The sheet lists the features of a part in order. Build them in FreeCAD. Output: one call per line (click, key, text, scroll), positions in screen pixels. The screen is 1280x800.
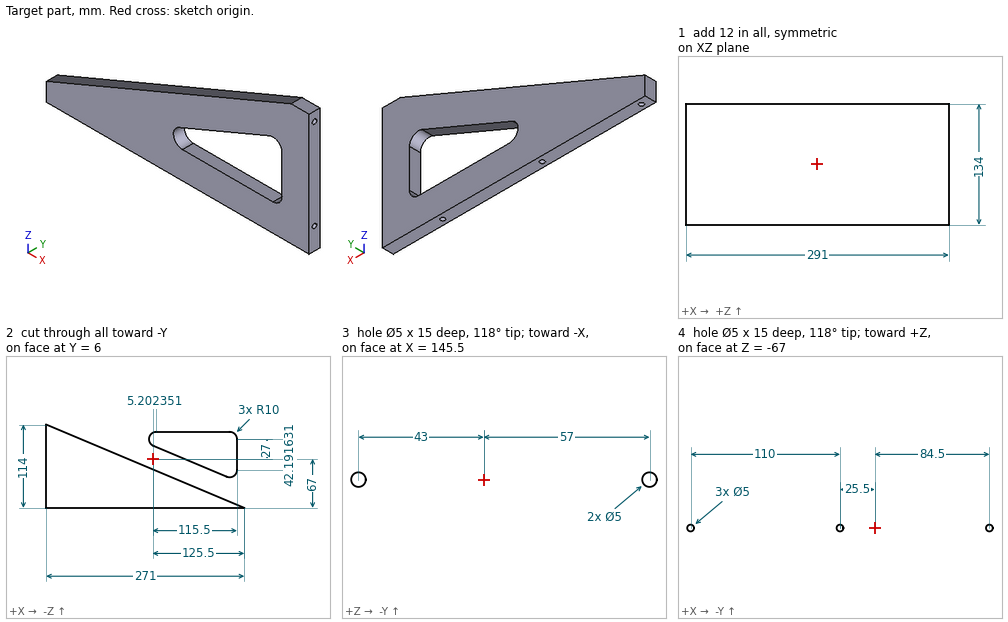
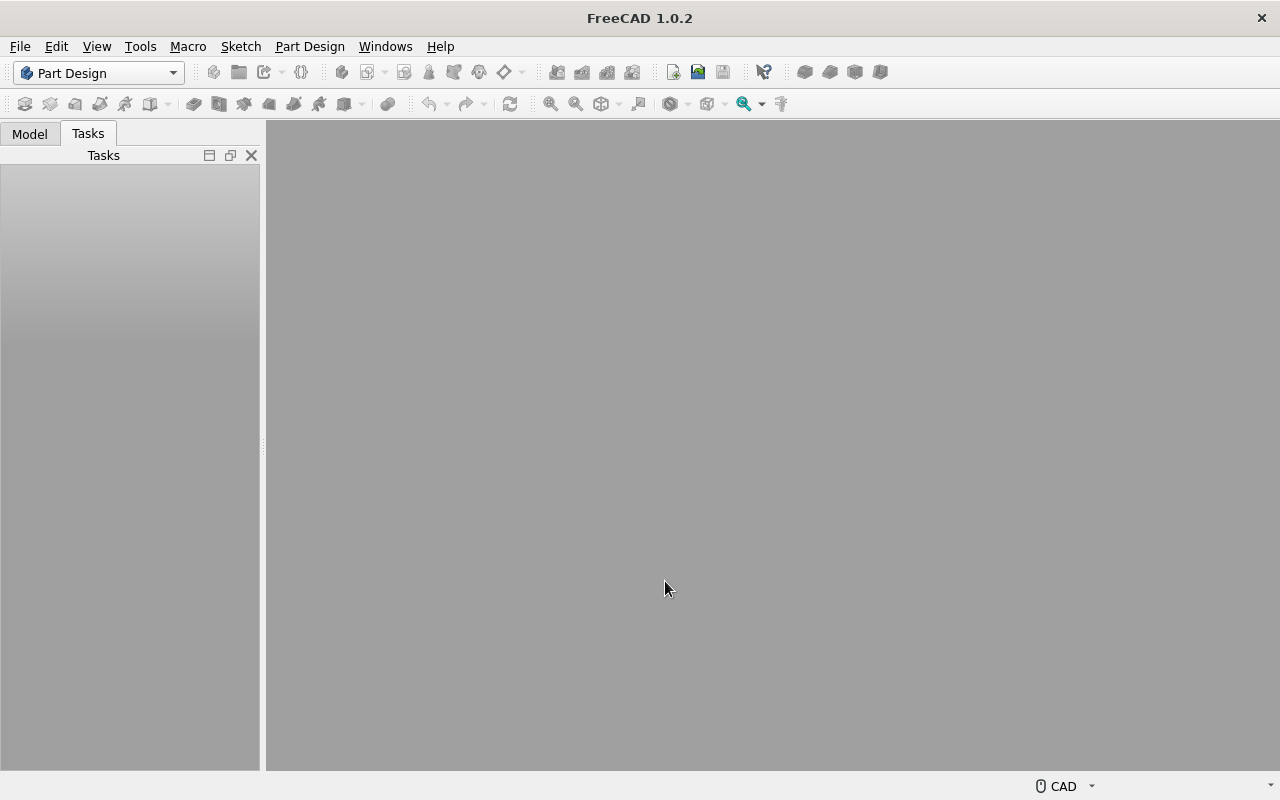
key(ctrl+n)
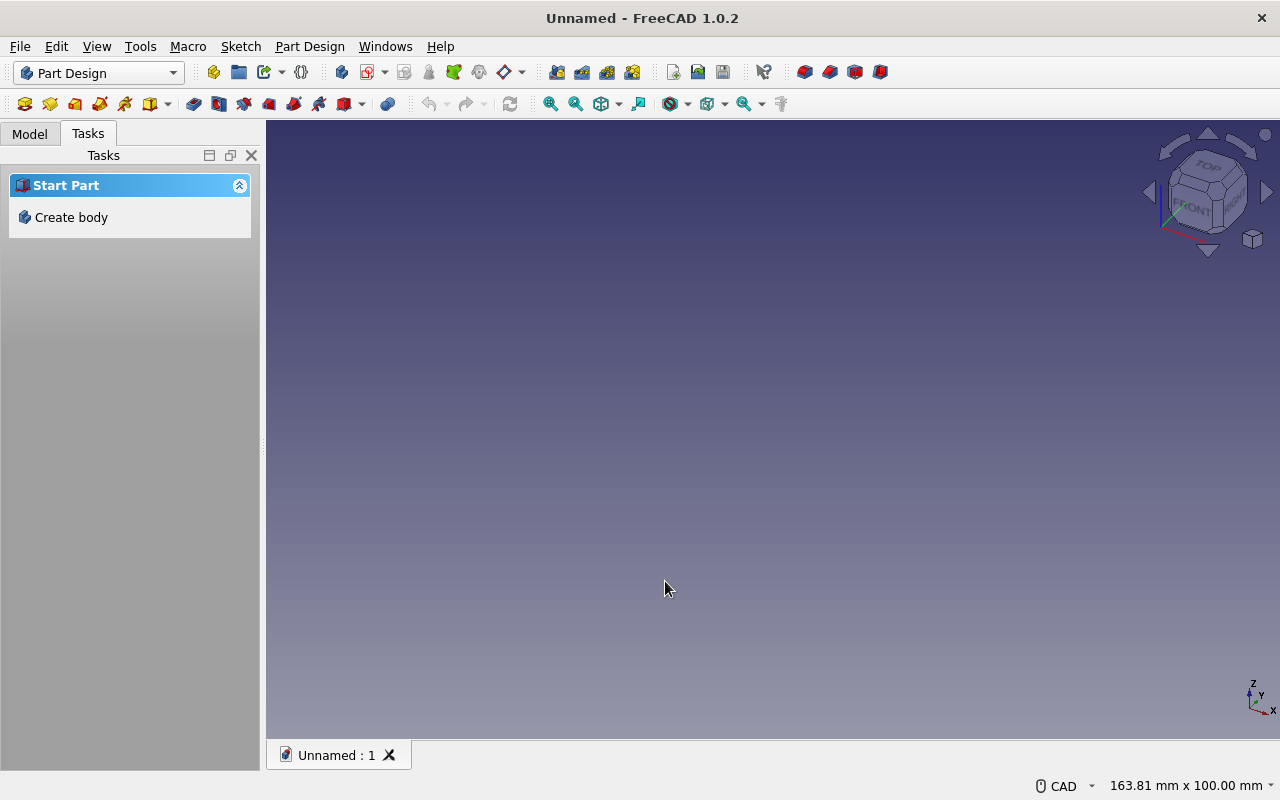
click(366, 72)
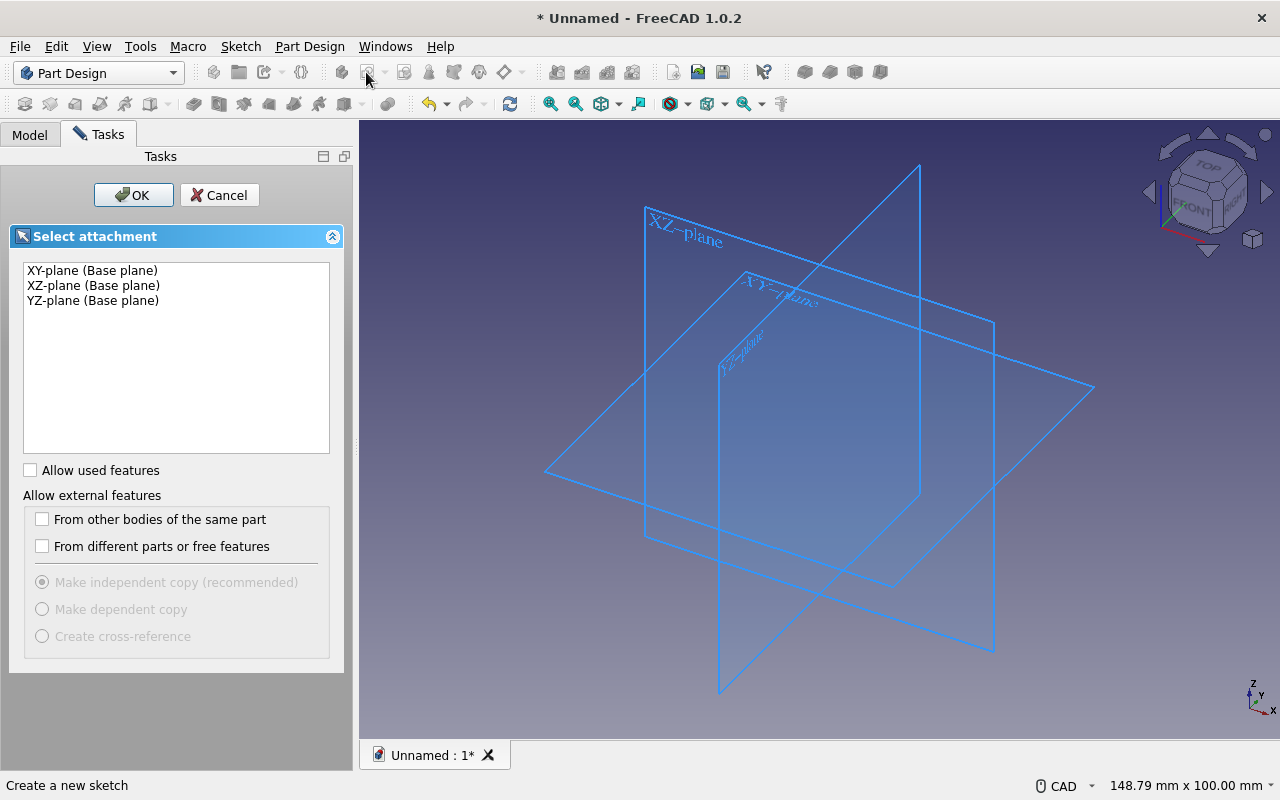
click(84, 286)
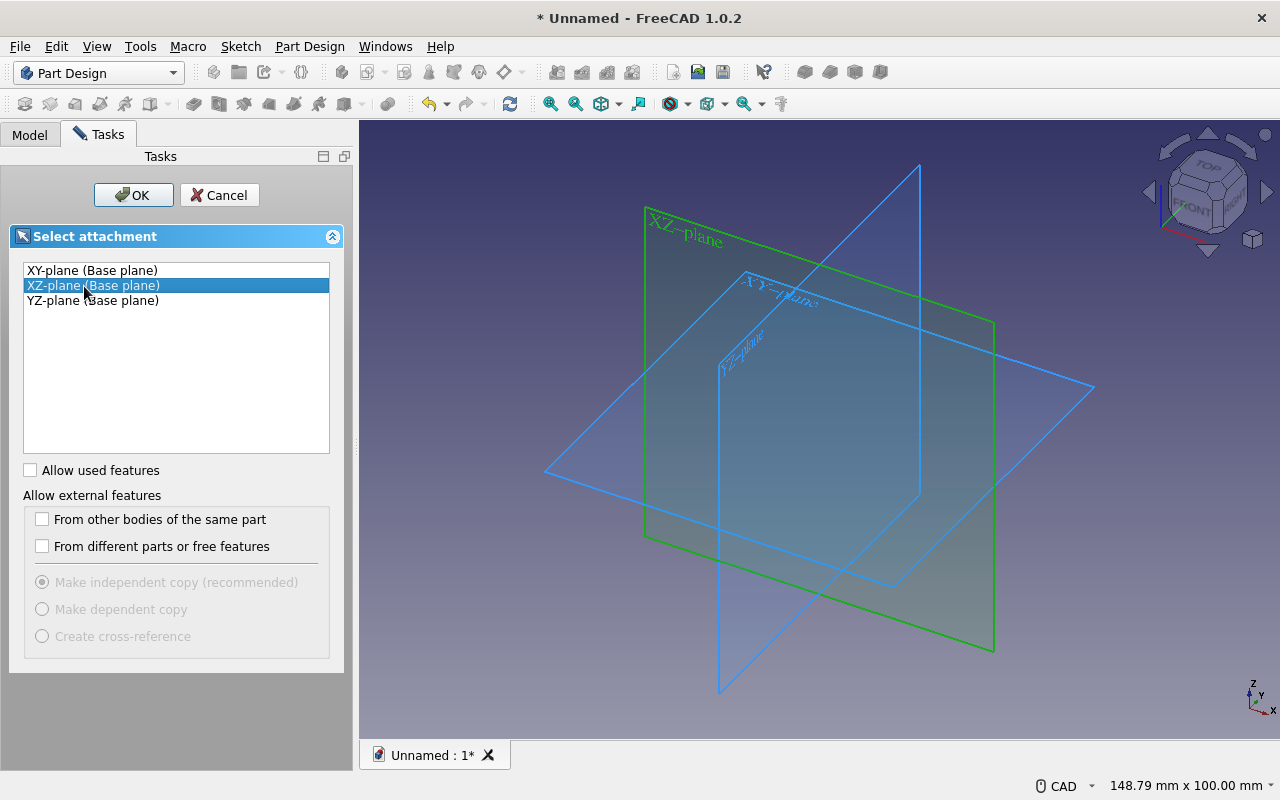
click(134, 195)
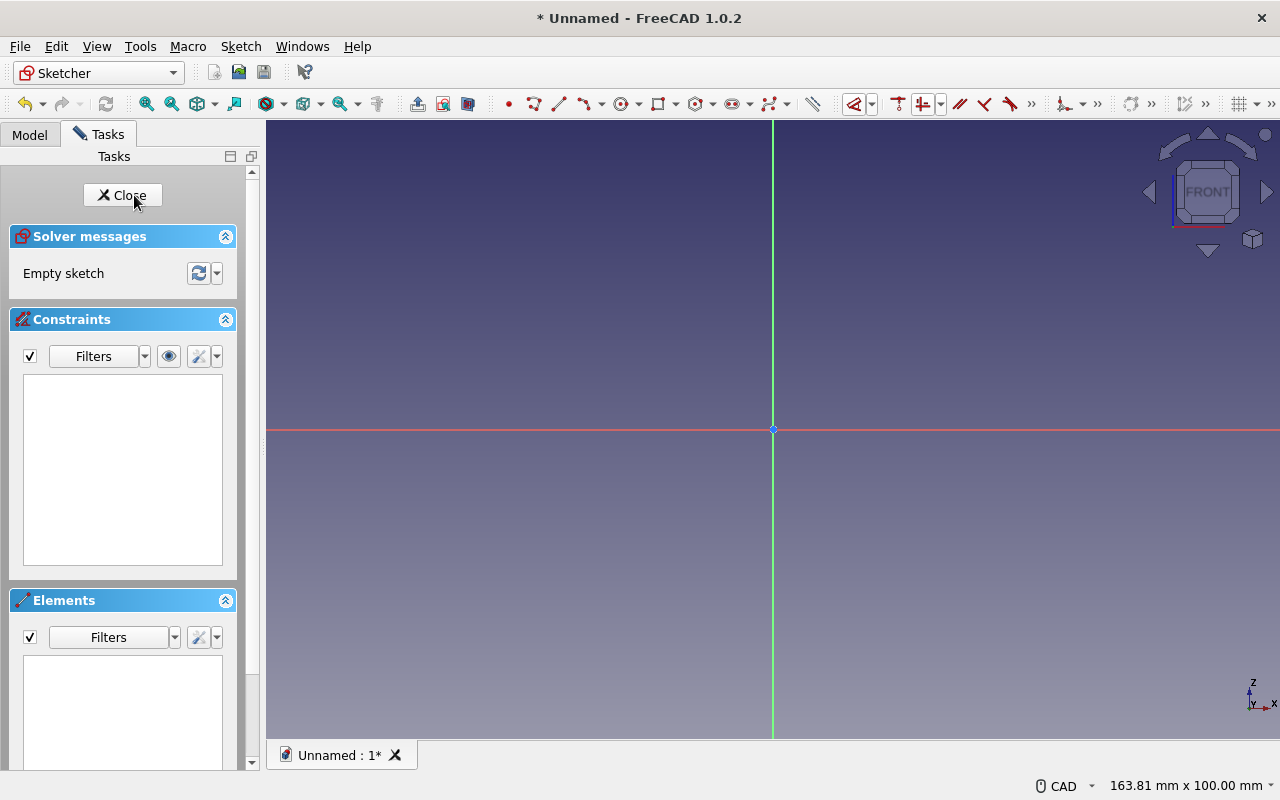
scroll(675, 429, down, 6)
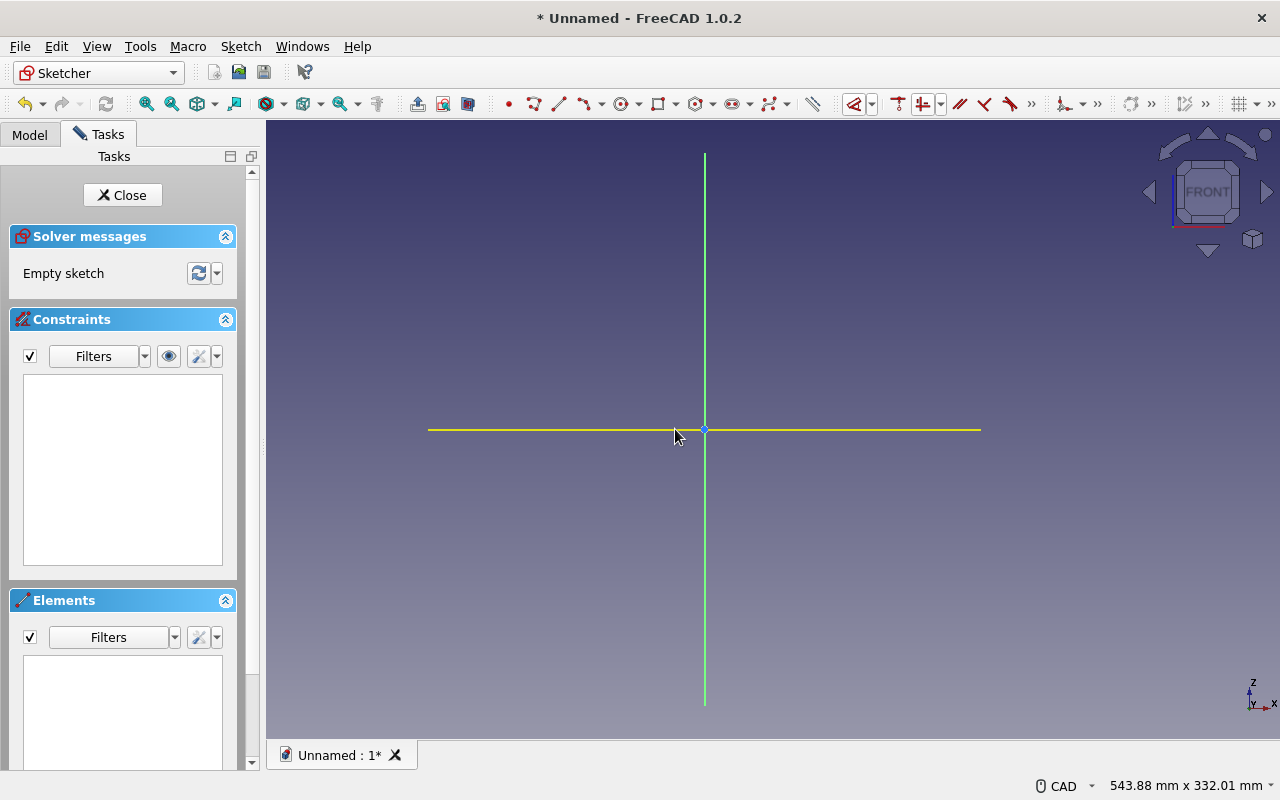
click(676, 104)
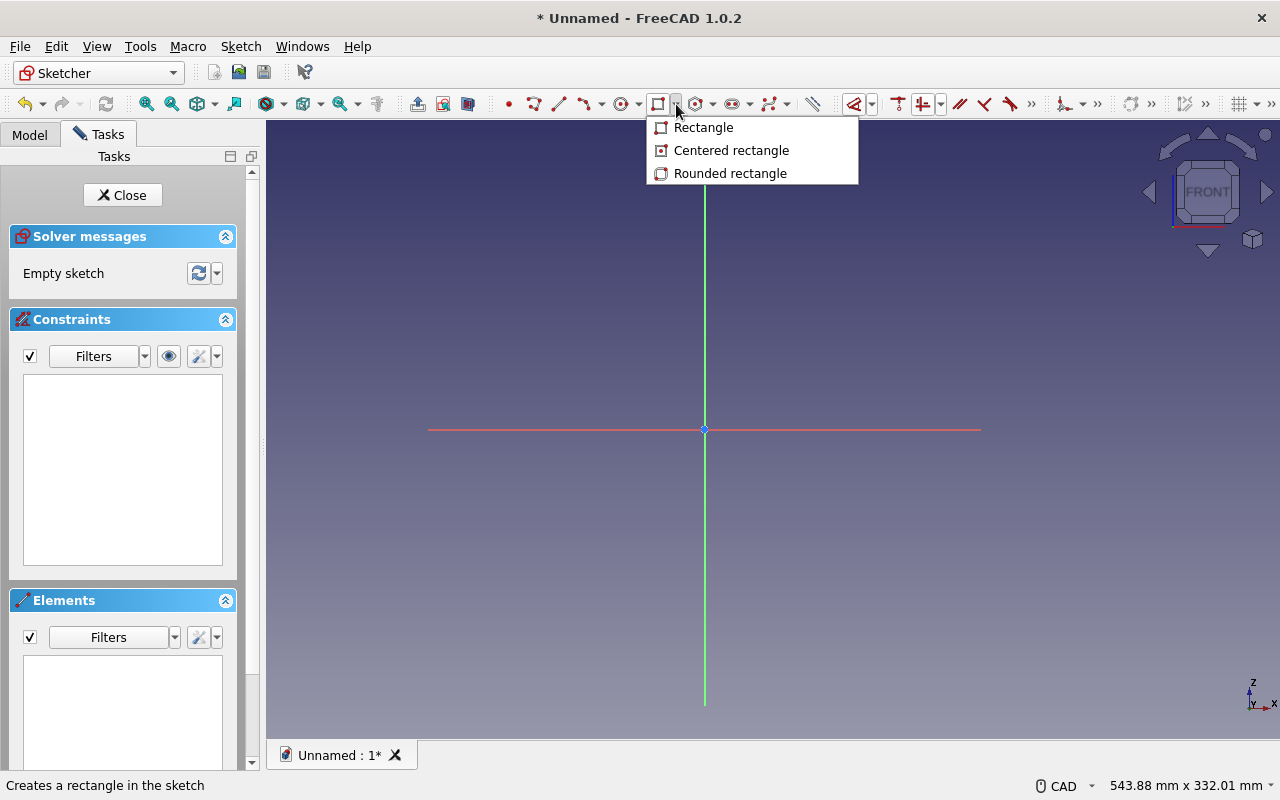
click(752, 150)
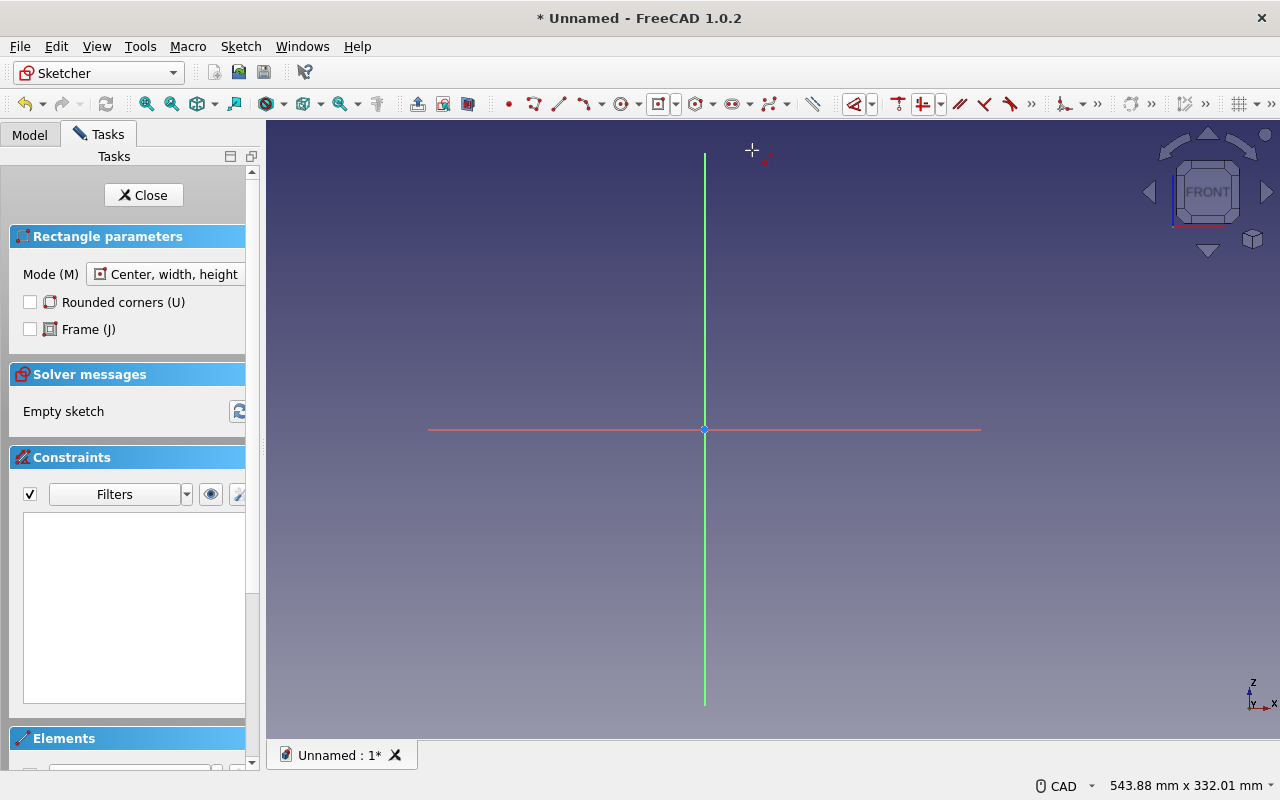
click(705, 430)
move(976, 305)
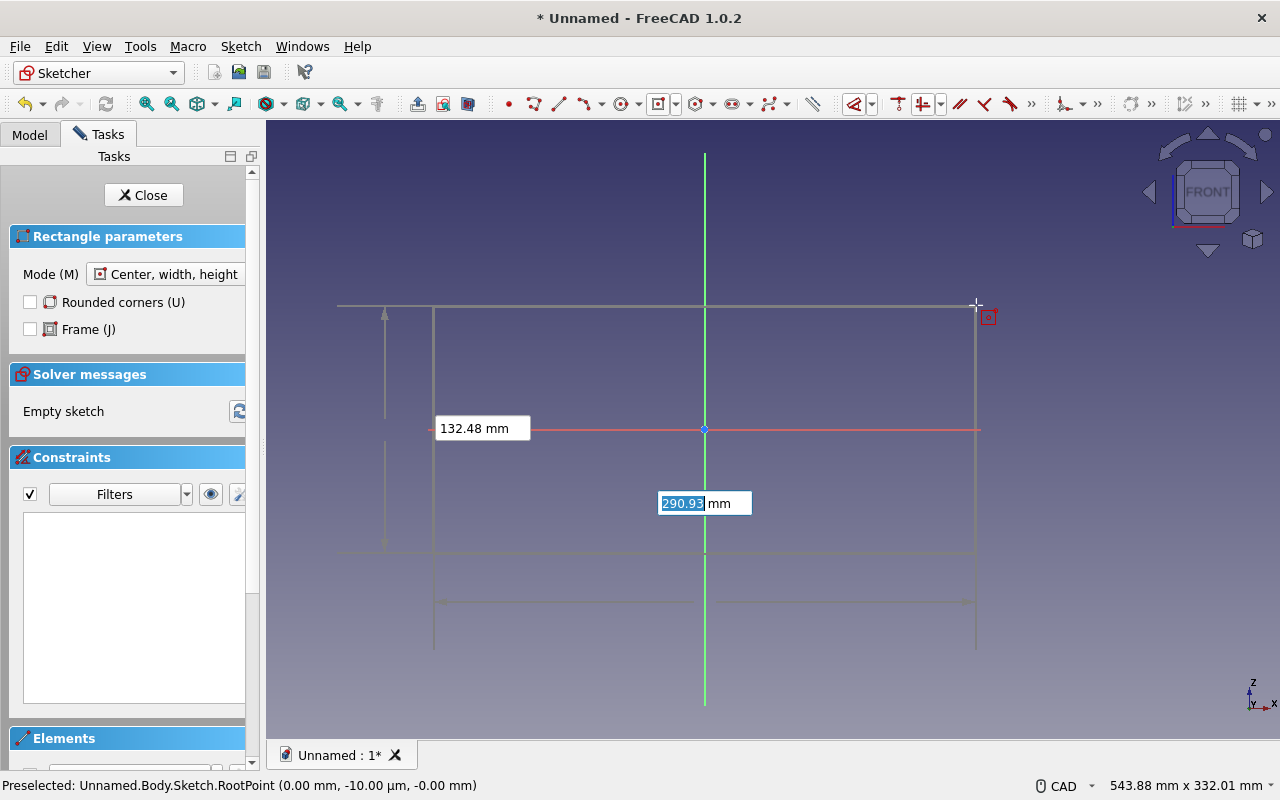
text(291)
key(Tab)
text(134)
key(Return)
key(Escape)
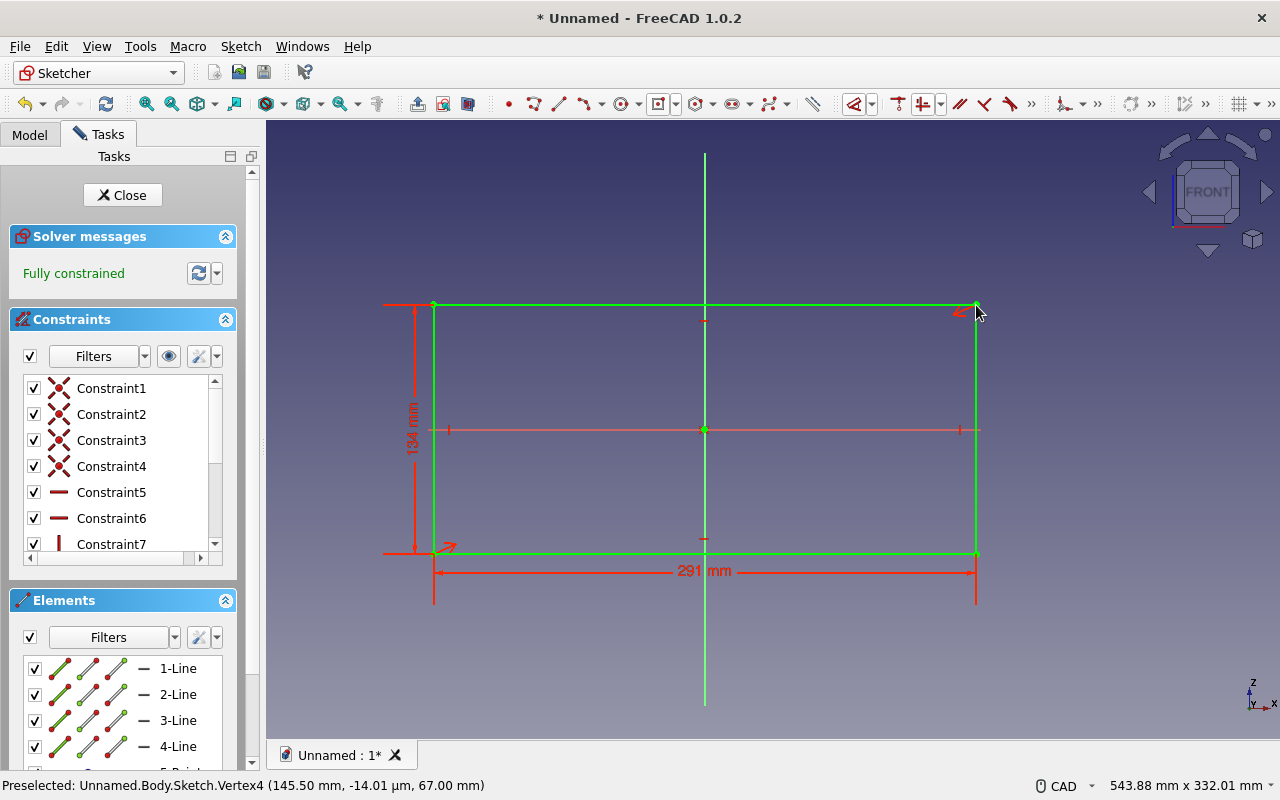
click(123, 195)